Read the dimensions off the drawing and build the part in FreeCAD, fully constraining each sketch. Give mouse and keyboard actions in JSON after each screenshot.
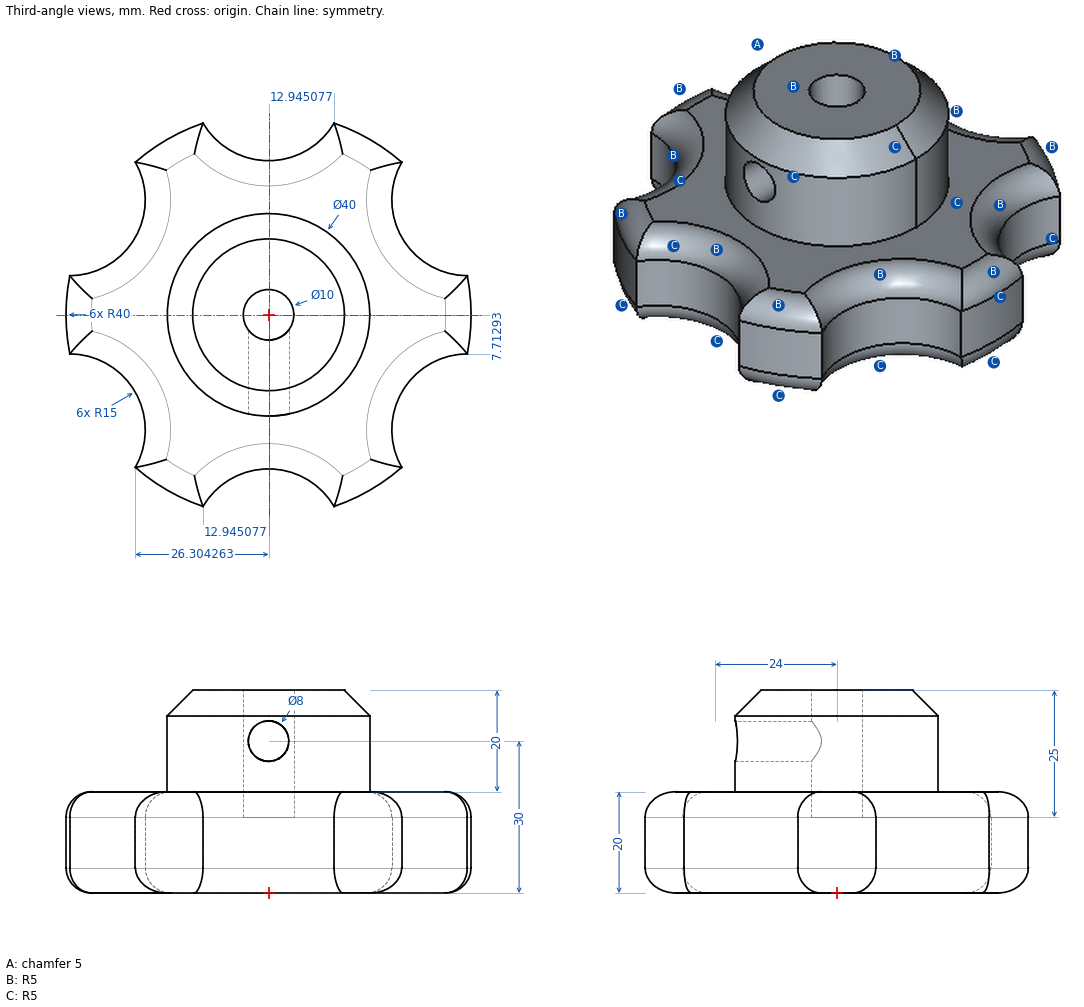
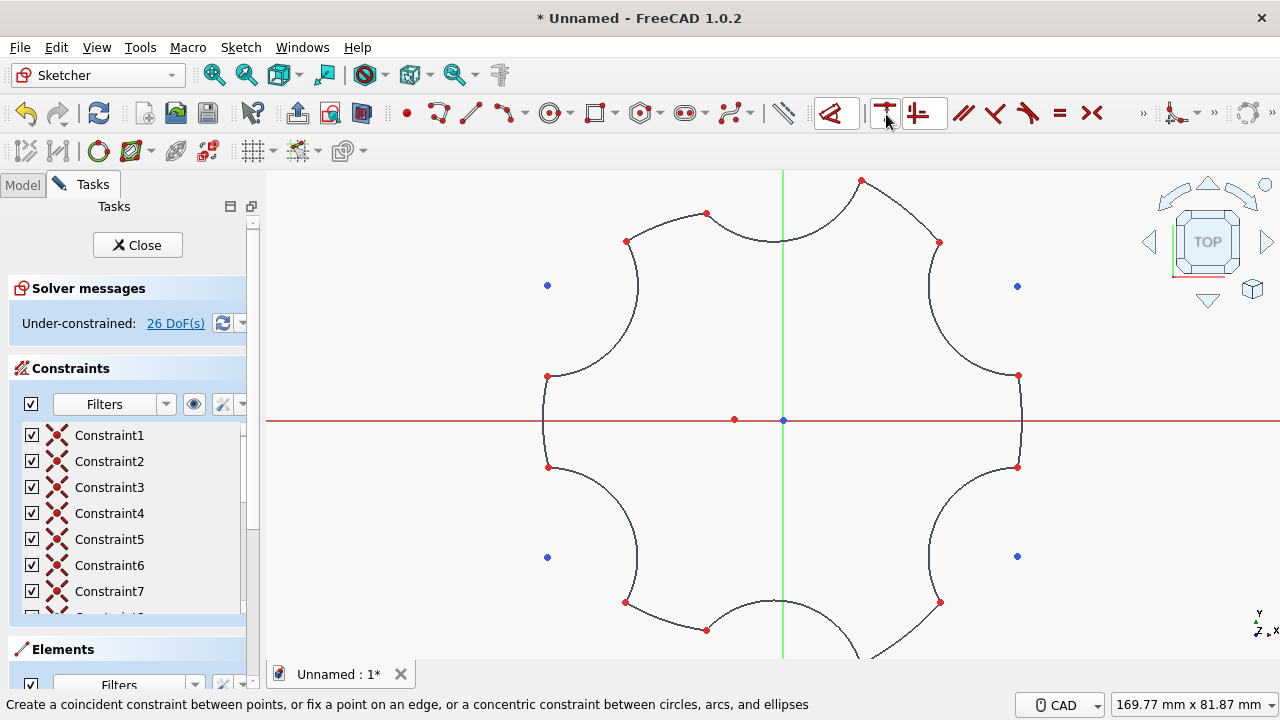
{"action": "left_click_drag", "start_coordinate": [725, 410], "coordinate": [793, 431]}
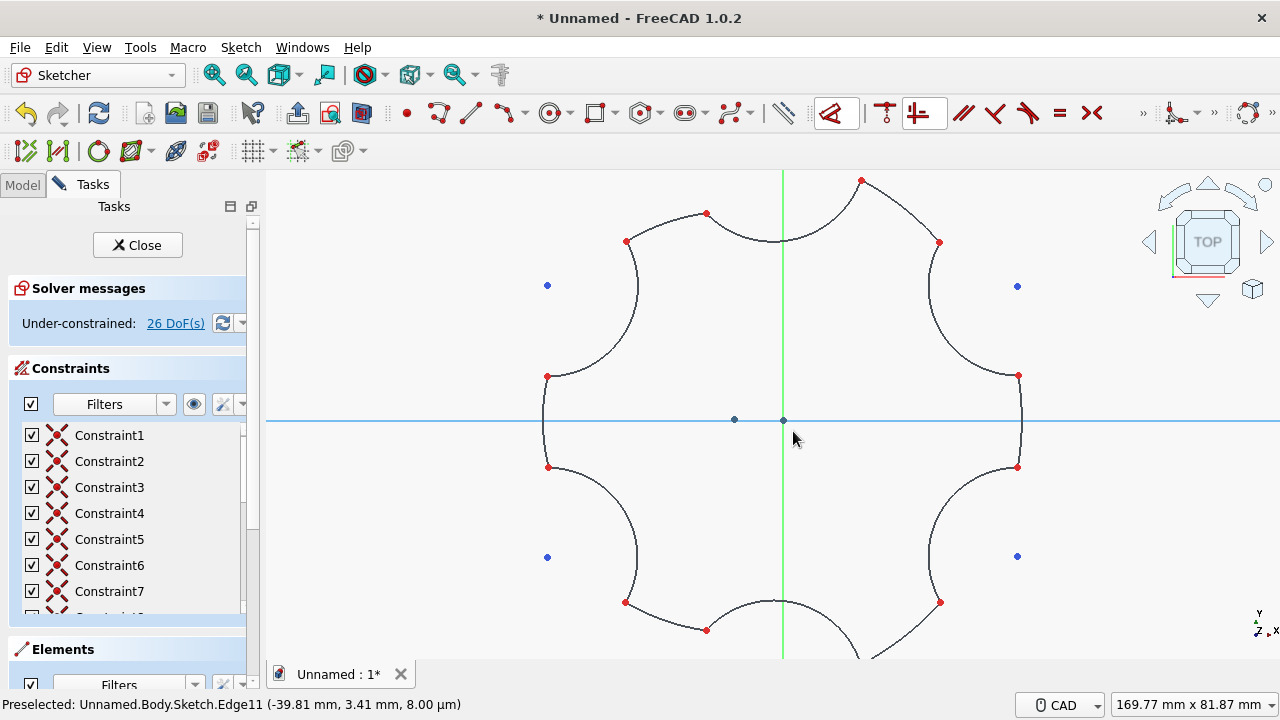
{"action": "left_click", "coordinate": [886, 114]}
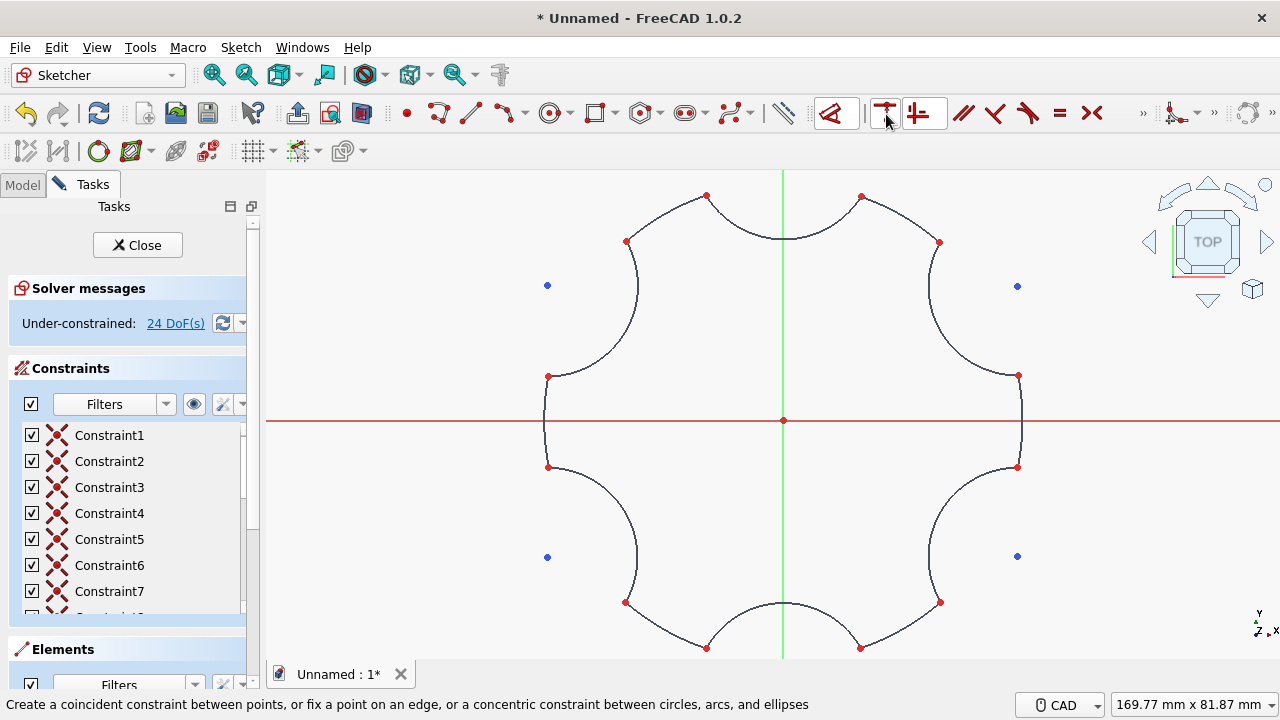
{"action": "left_click", "coordinate": [648, 619]}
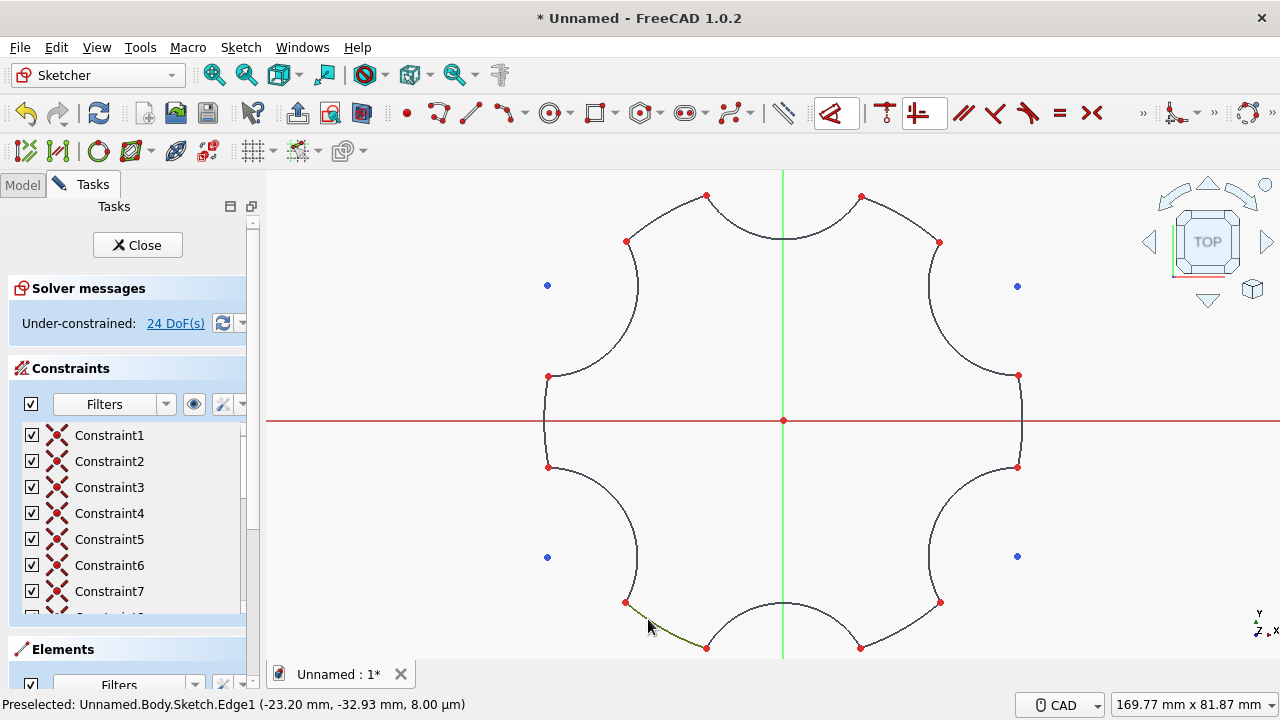
{"action": "left_click", "coordinate": [919, 619]}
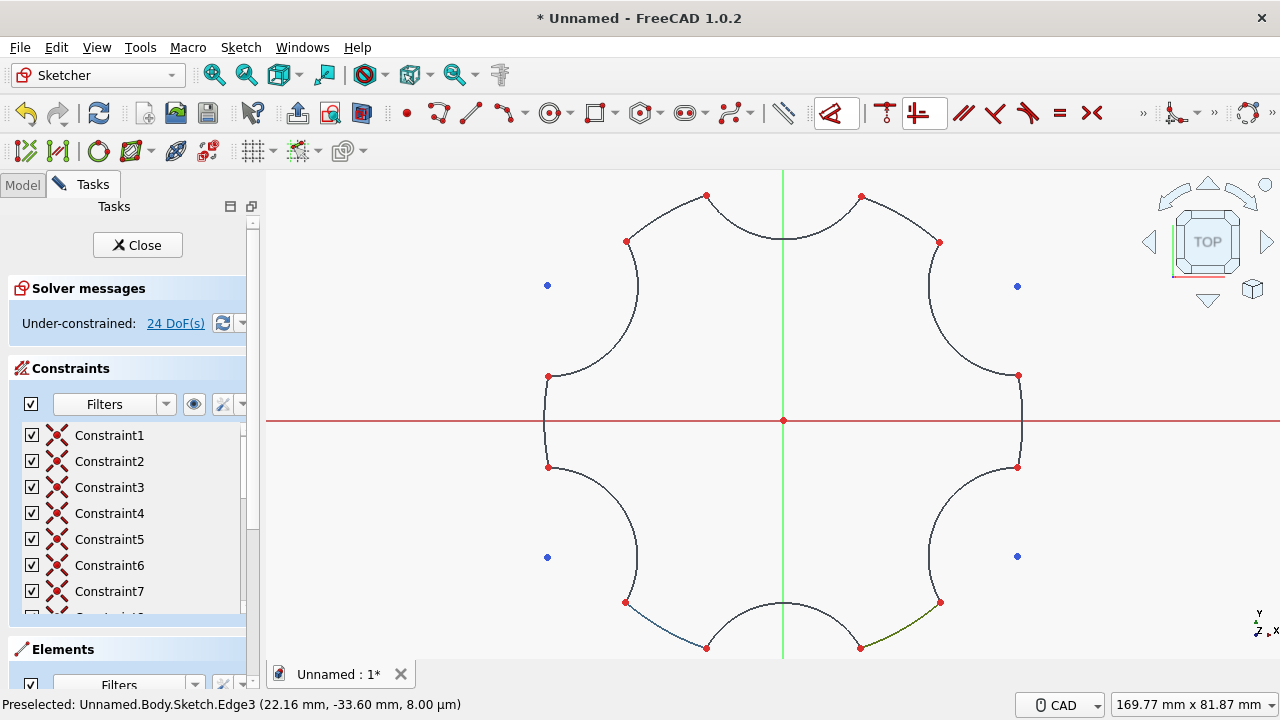
{"action": "left_click", "coordinate": [1022, 440]}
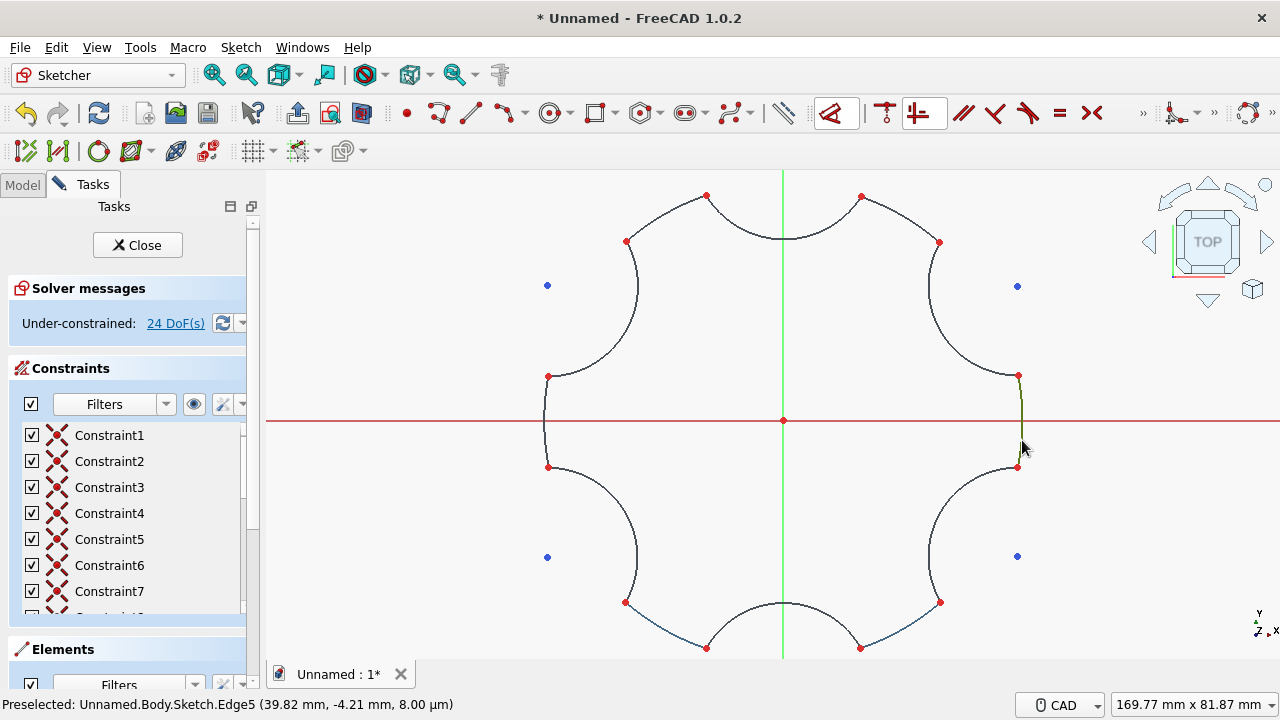
{"action": "left_click", "coordinate": [918, 226]}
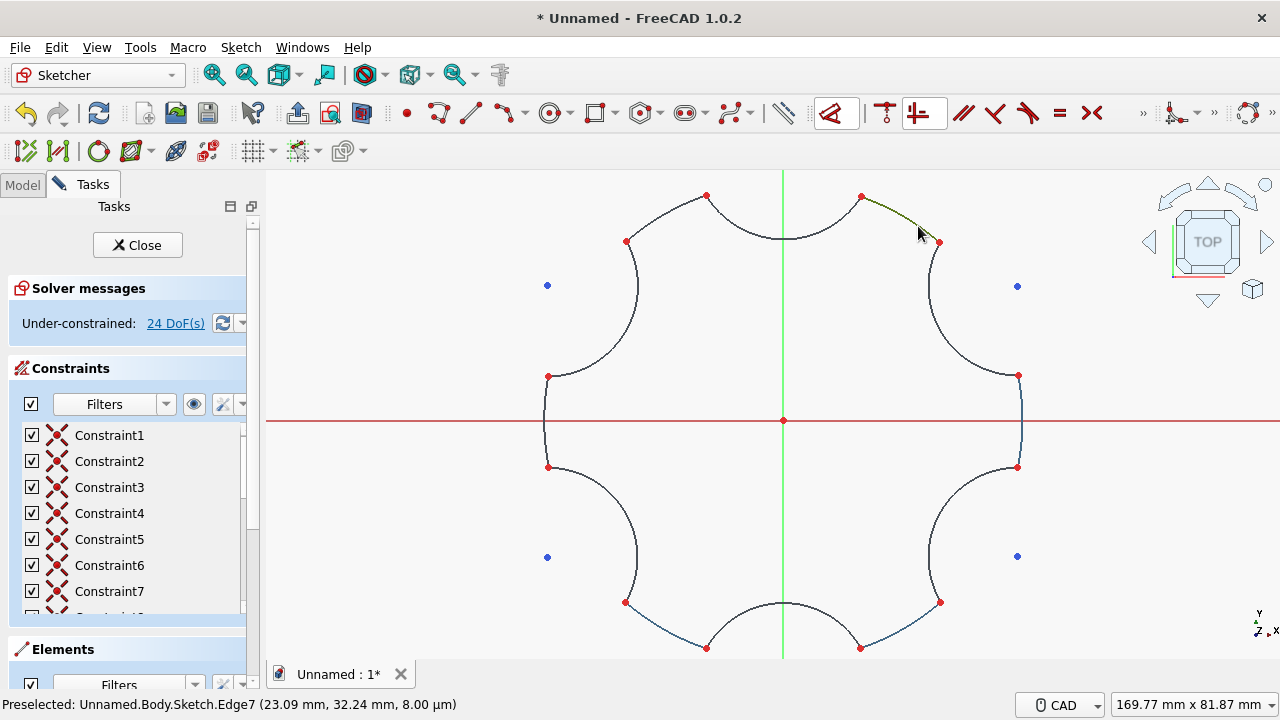
{"action": "left_click", "coordinate": [680, 206]}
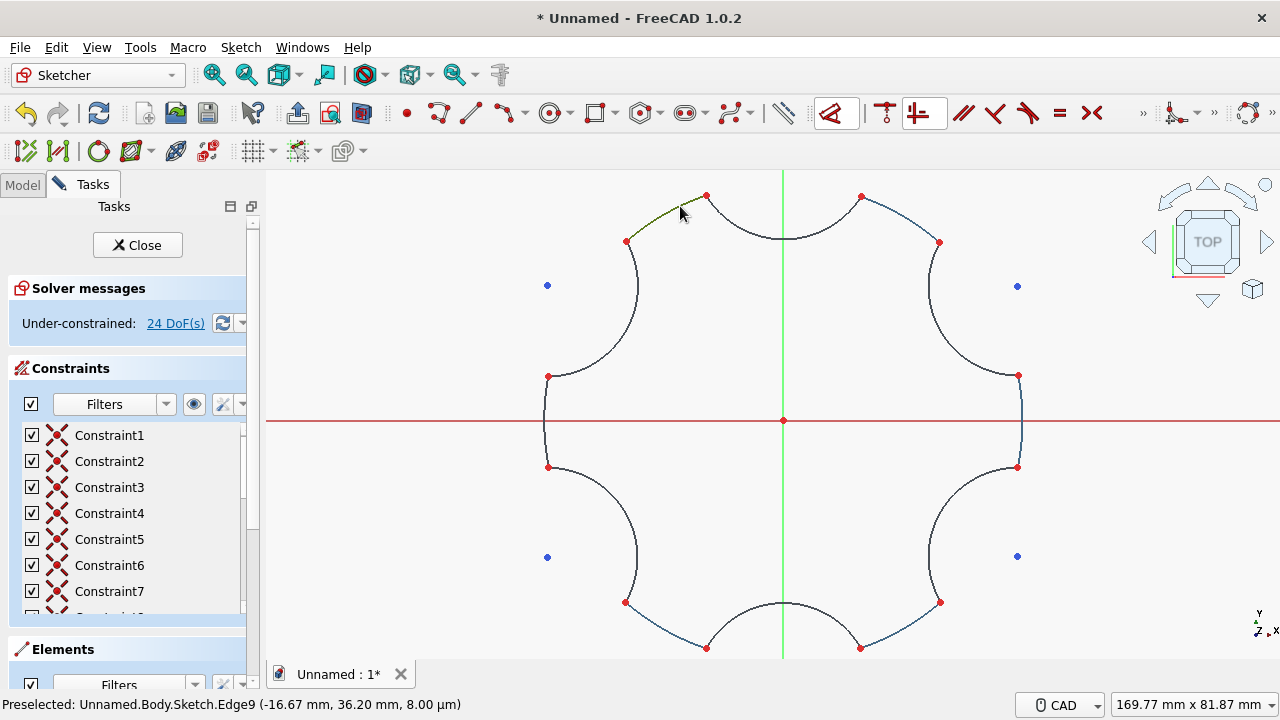
{"action": "left_click", "coordinate": [545, 404]}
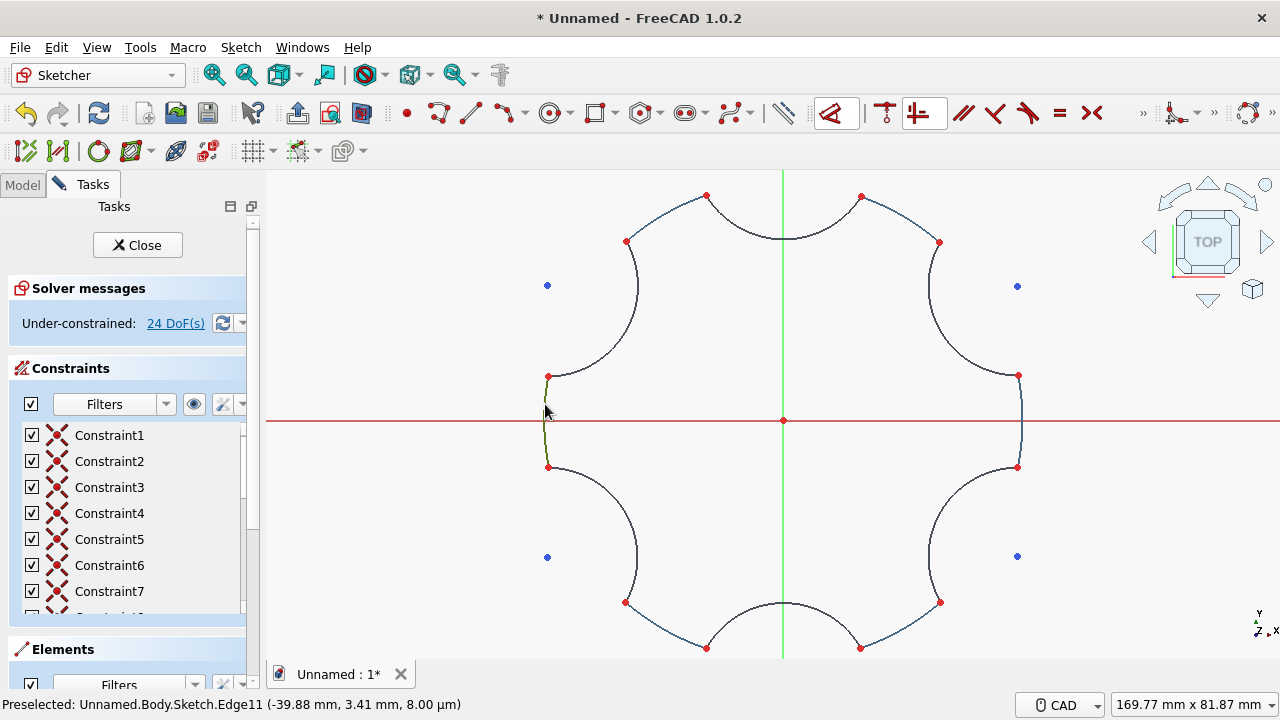
{"action": "left_click", "coordinate": [1060, 114]}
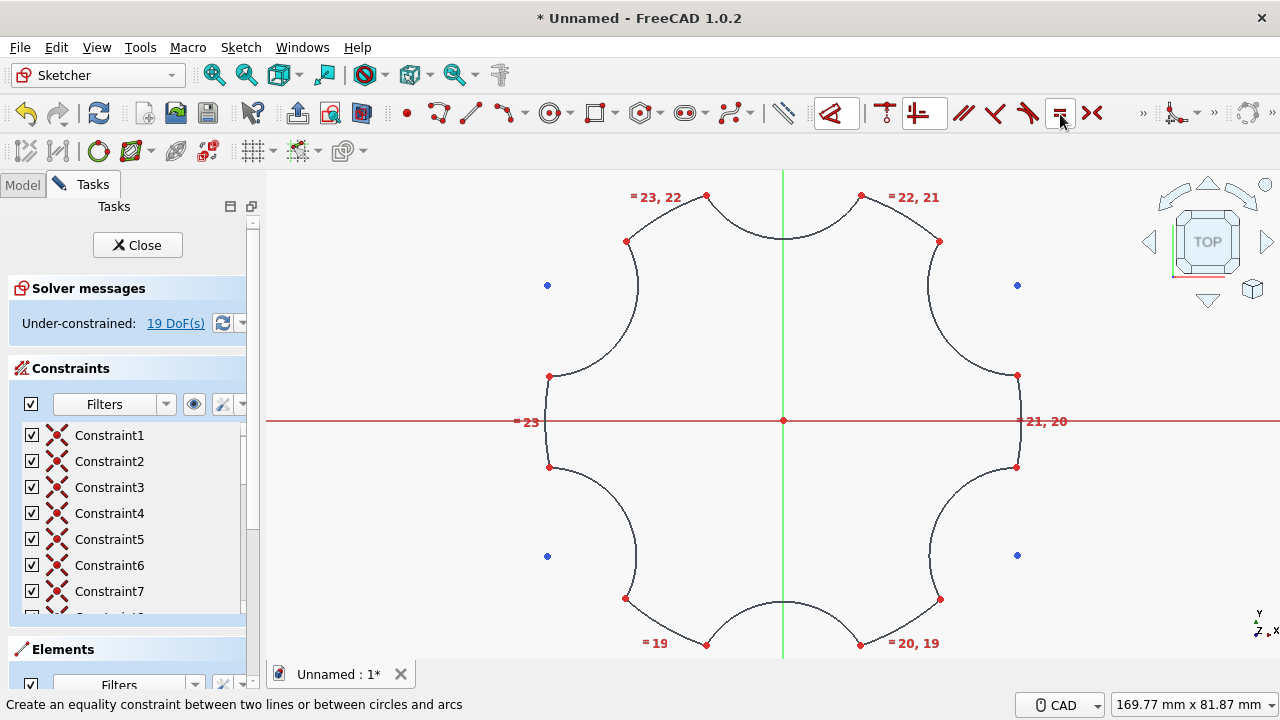
{"action": "left_click", "coordinate": [820, 609]}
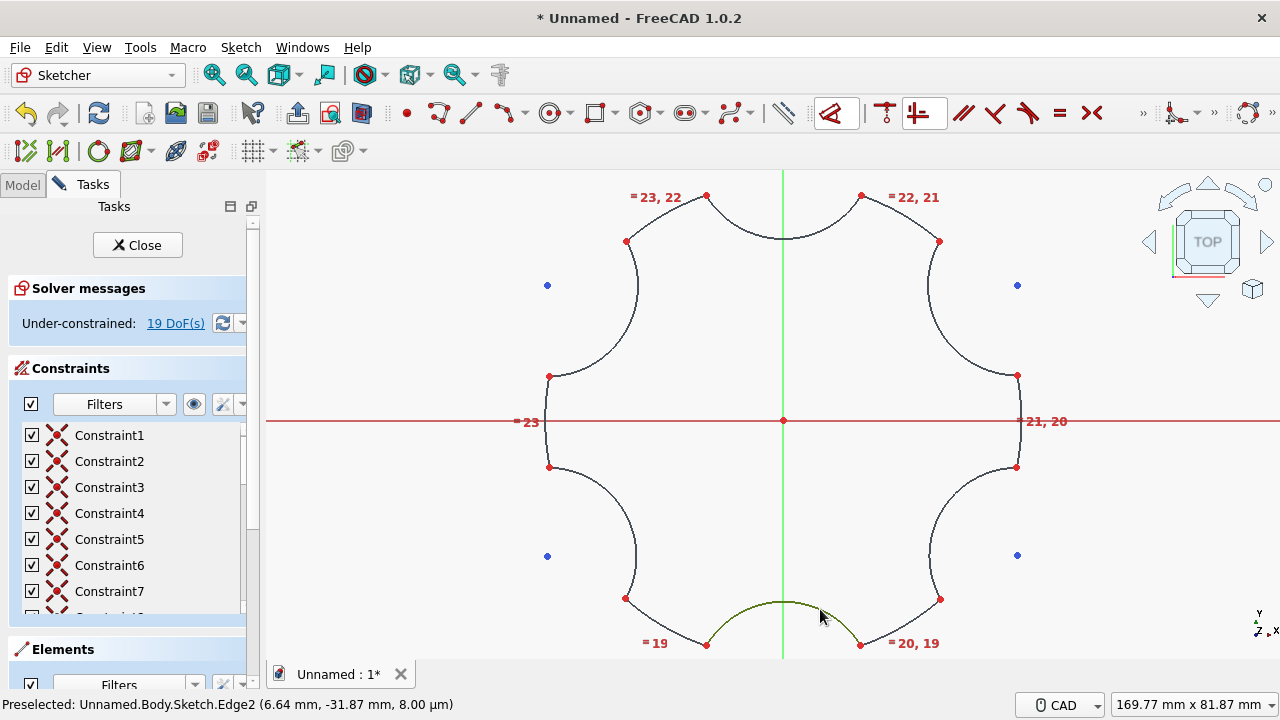
{"action": "left_click", "coordinate": [966, 485]}